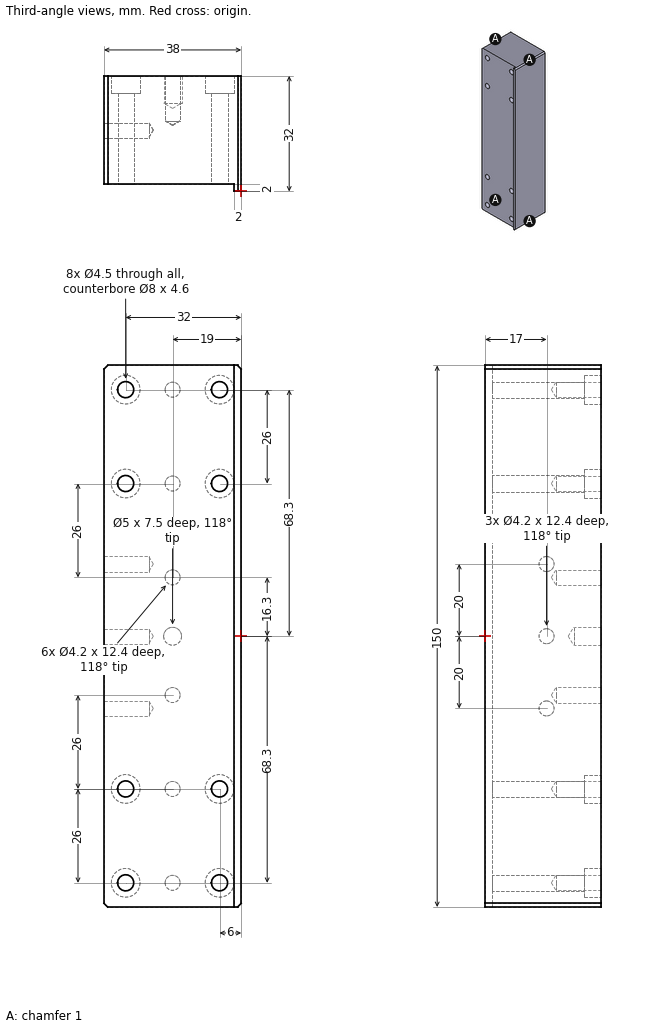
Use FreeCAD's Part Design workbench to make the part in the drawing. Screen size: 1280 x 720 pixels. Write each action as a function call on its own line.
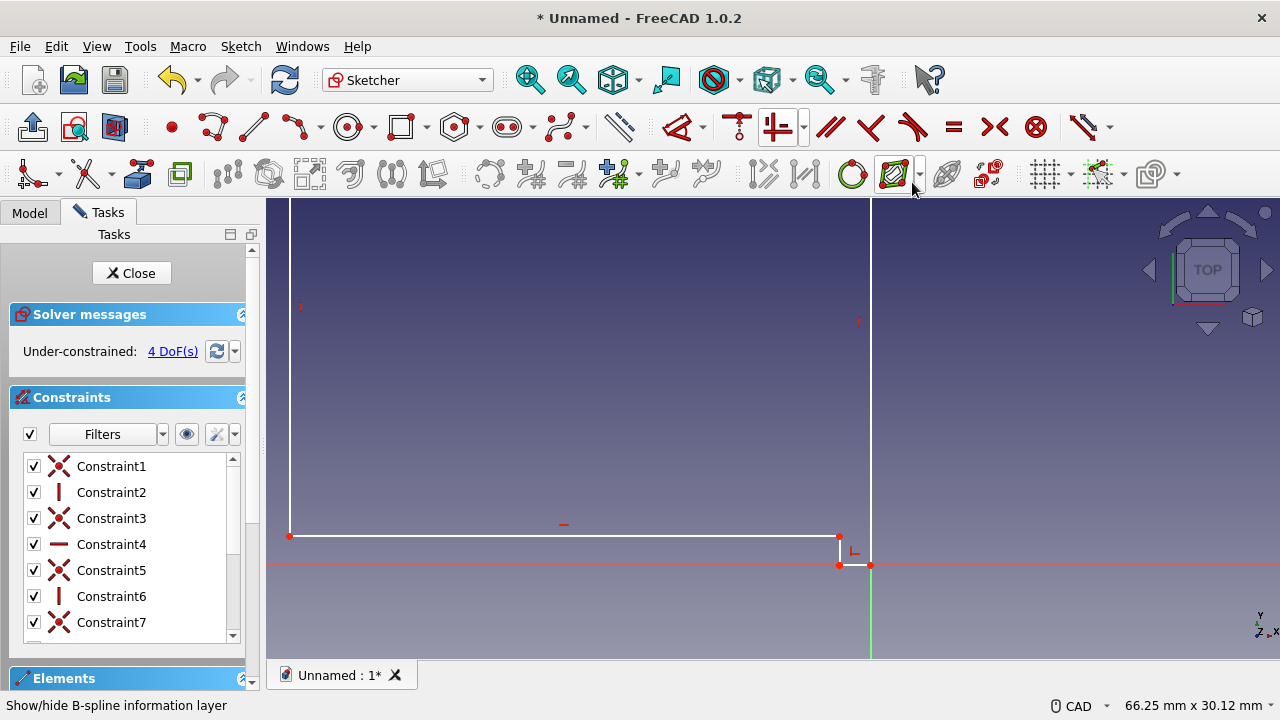
key(d)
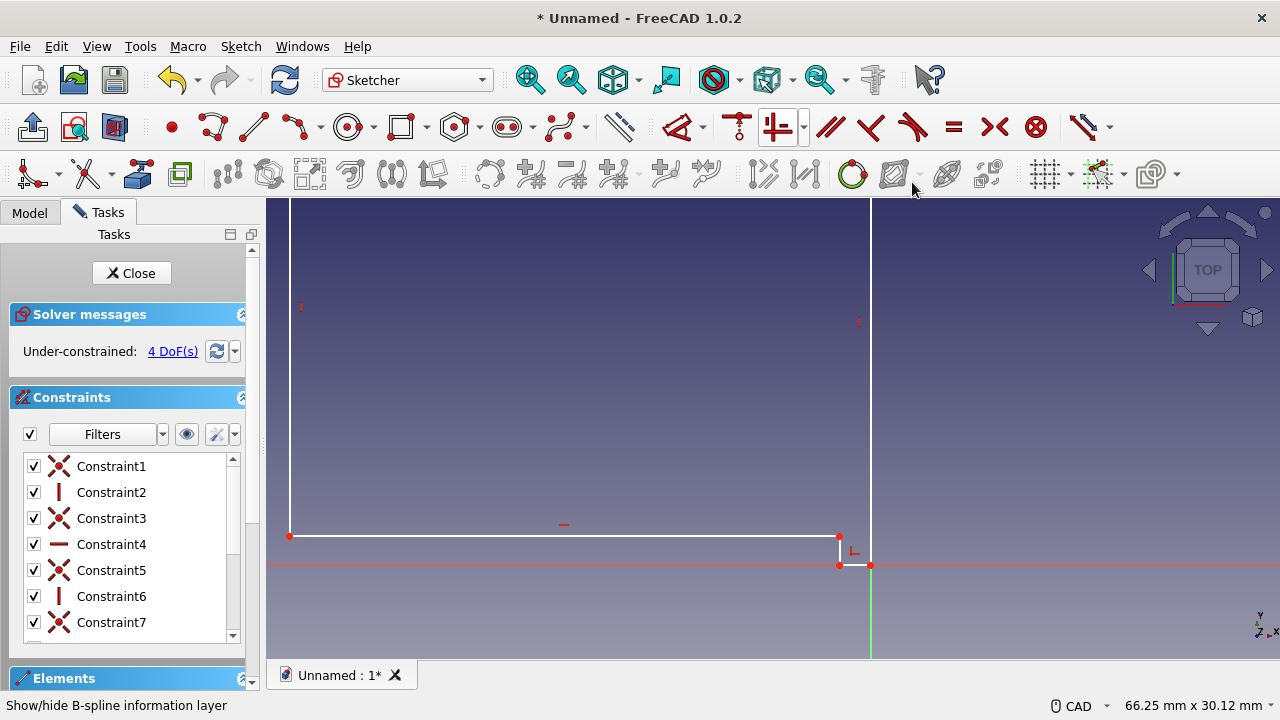
scroll(840, 548, up, 2)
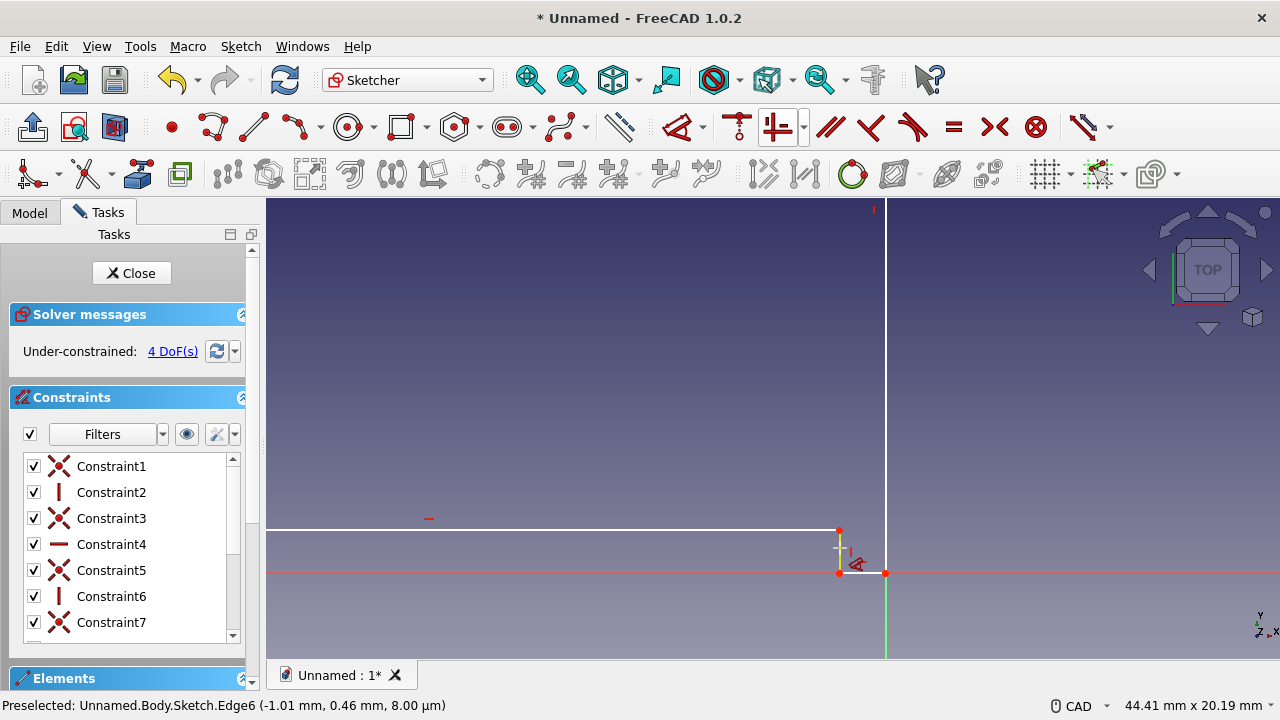
click(840, 548)
click(806, 552)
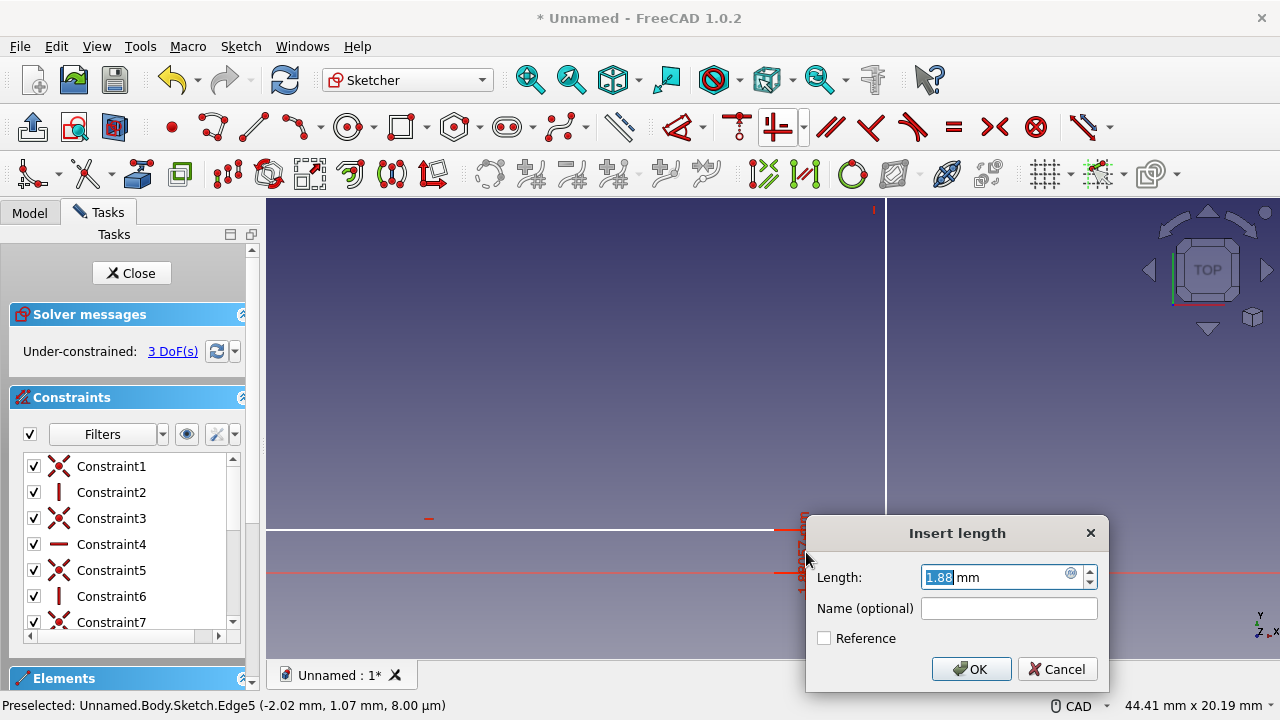
text(2)
key(Return)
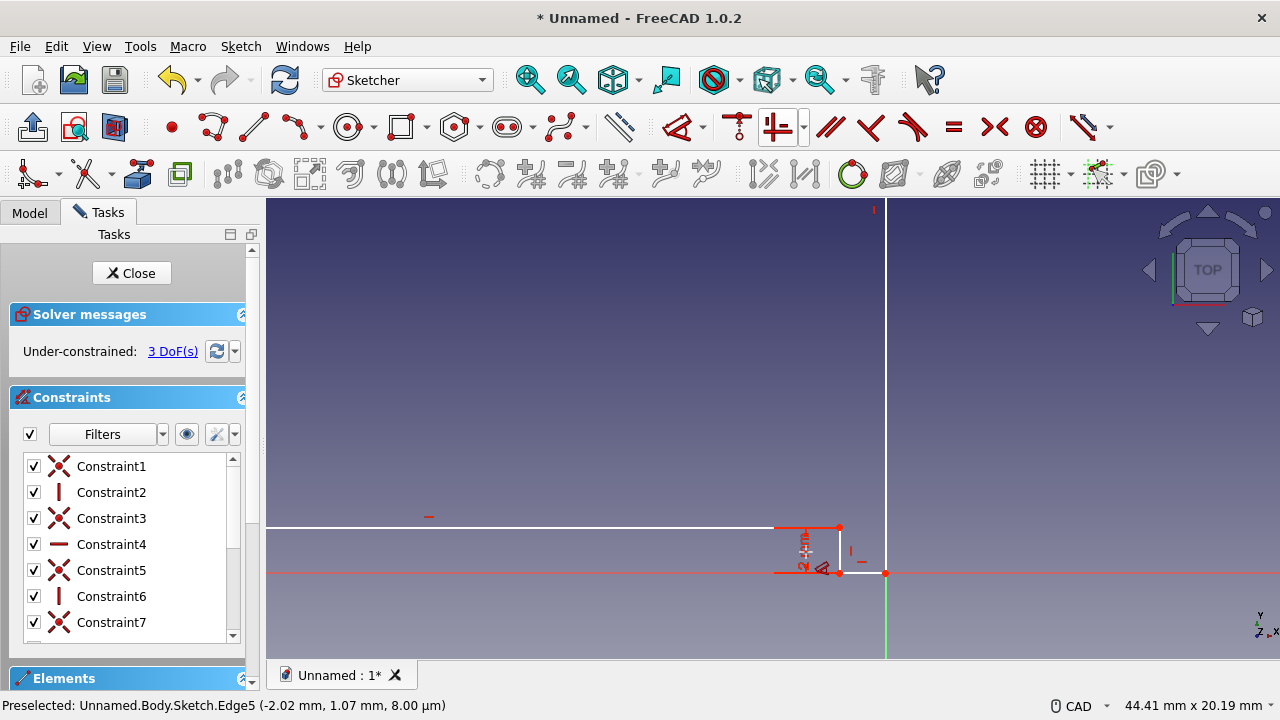
click(853, 573)
click(863, 607)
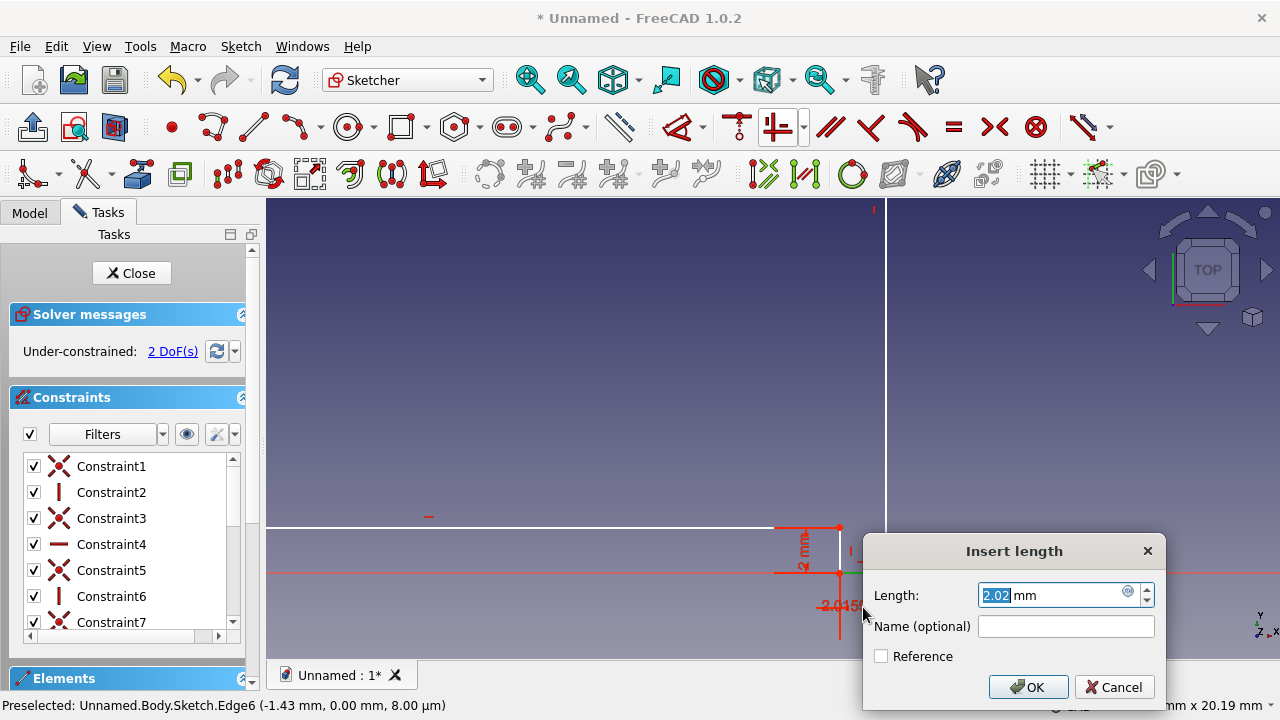
text(2)
key(Return)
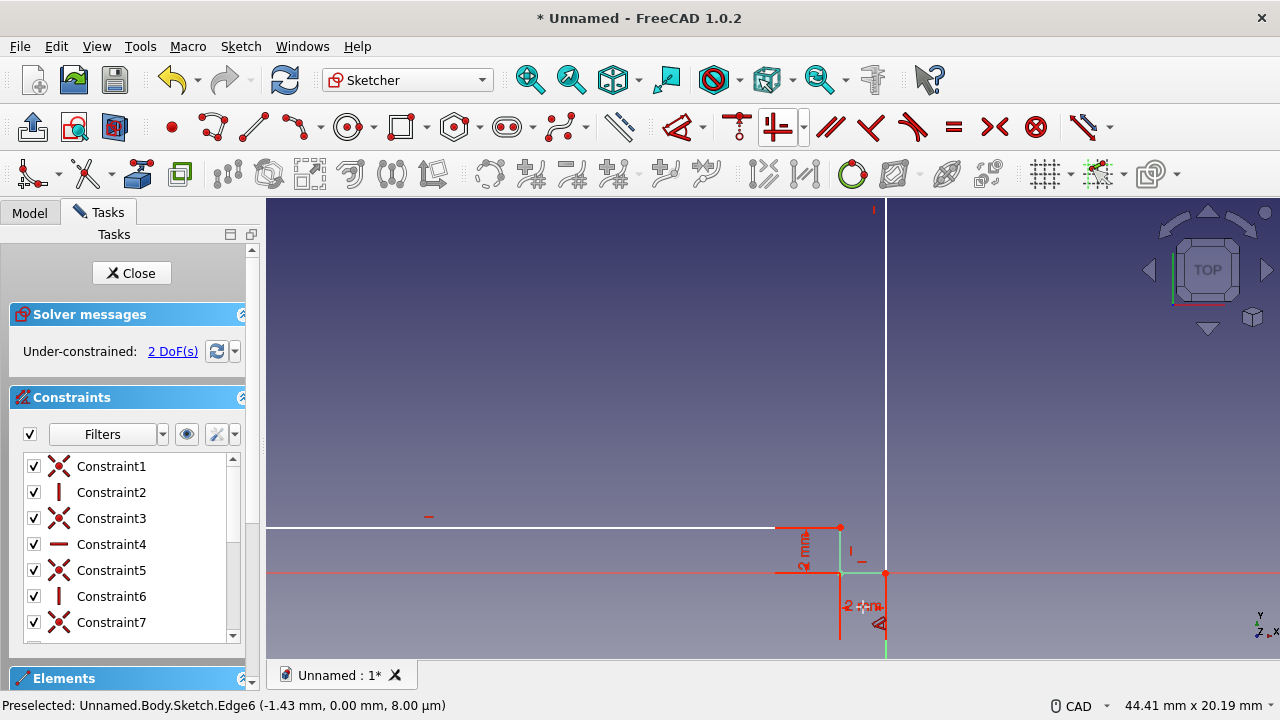
click(886, 355)
click(920, 400)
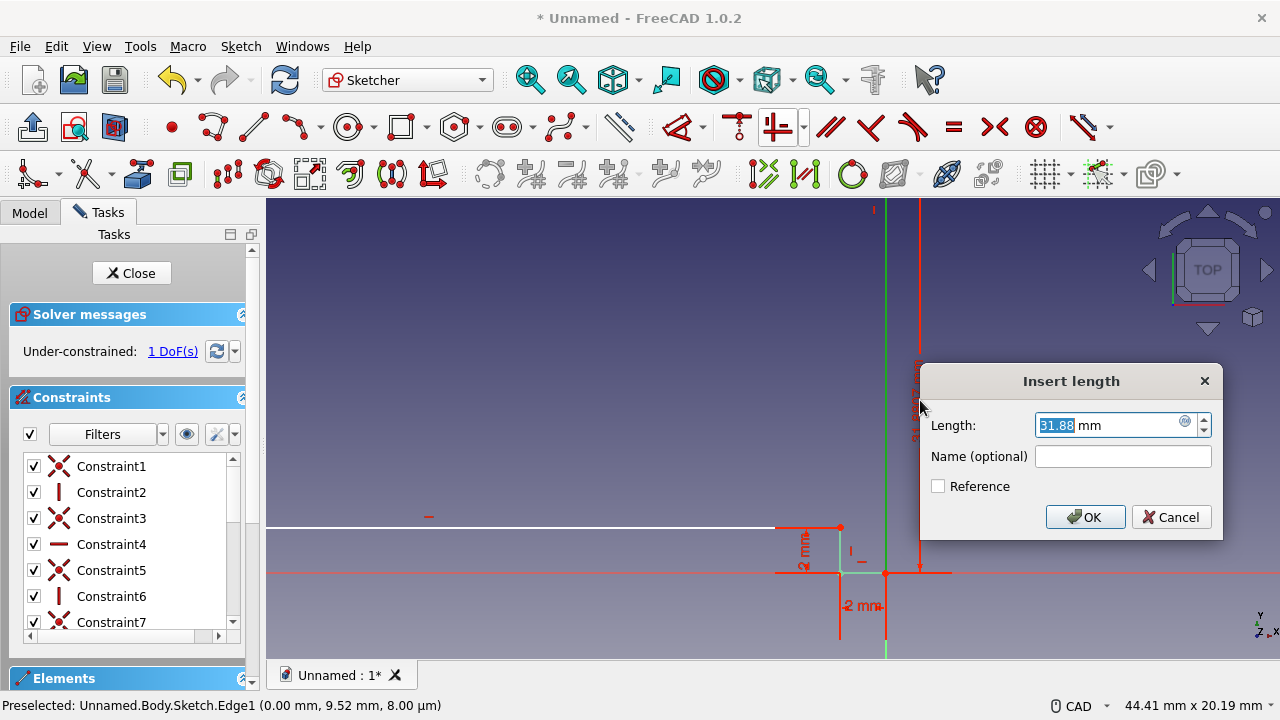
text(32)
key(Return)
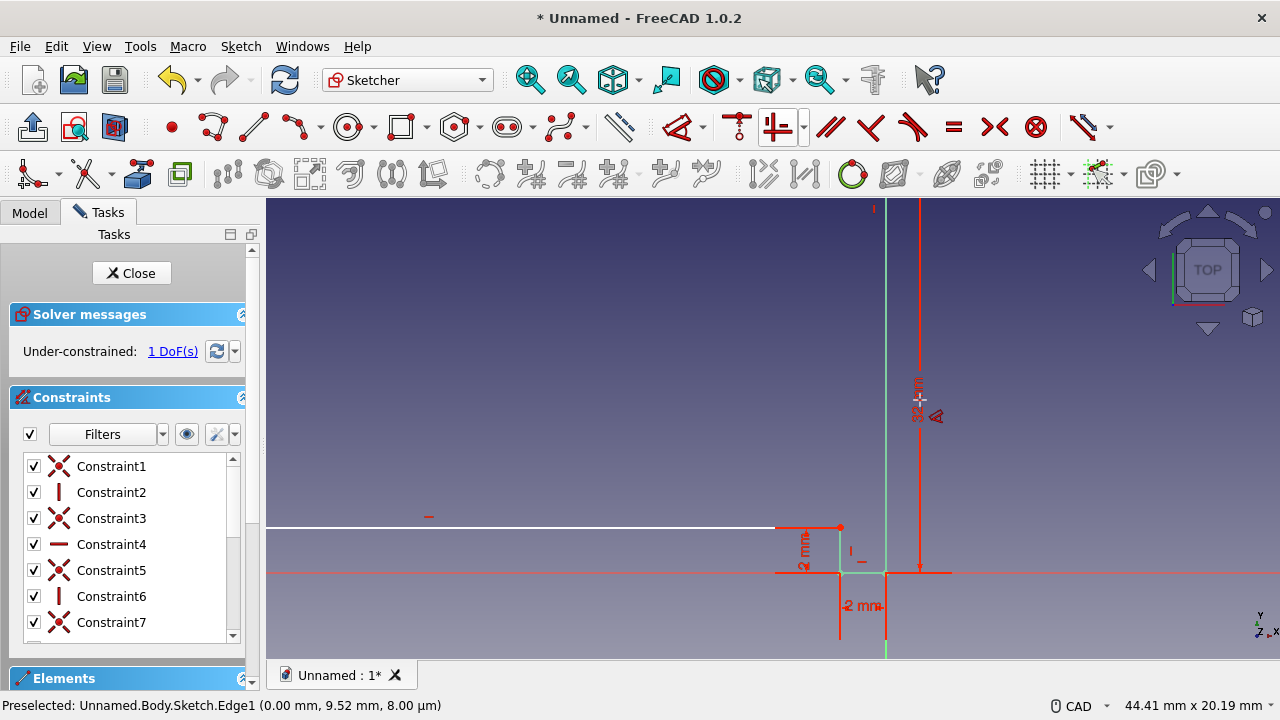
scroll(852, 557, down, 5)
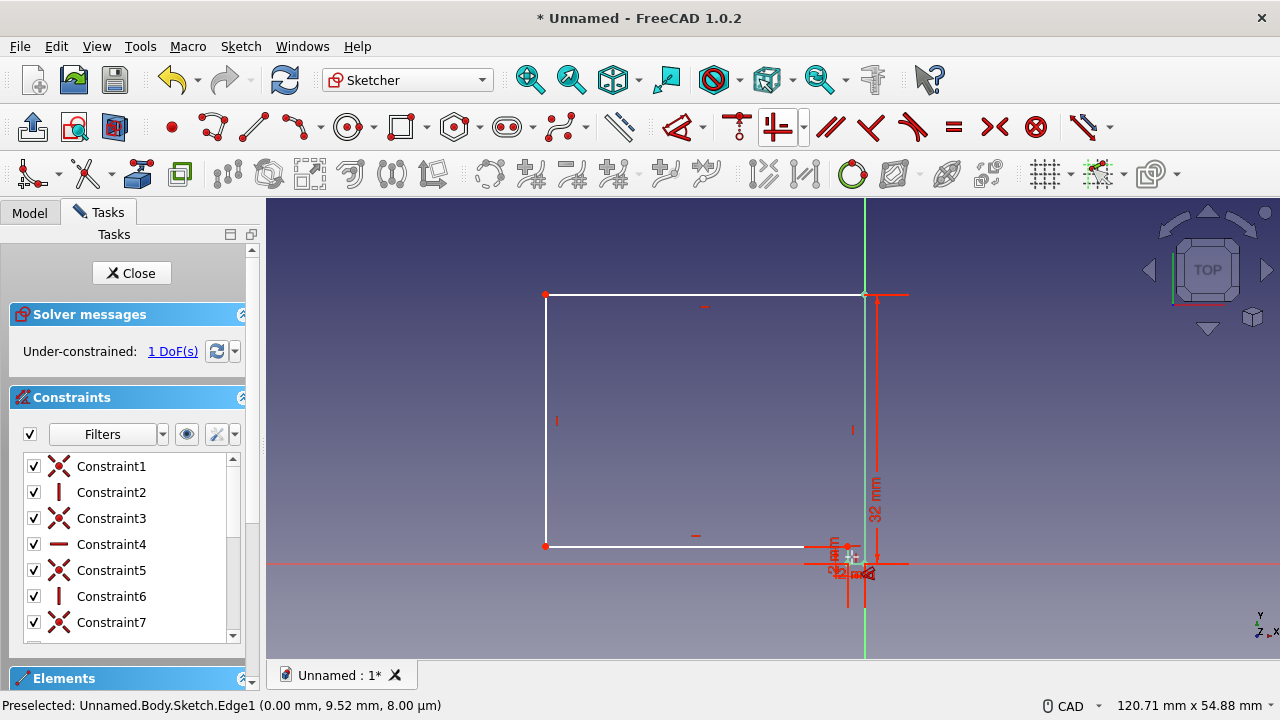
click(769, 295)
click(705, 261)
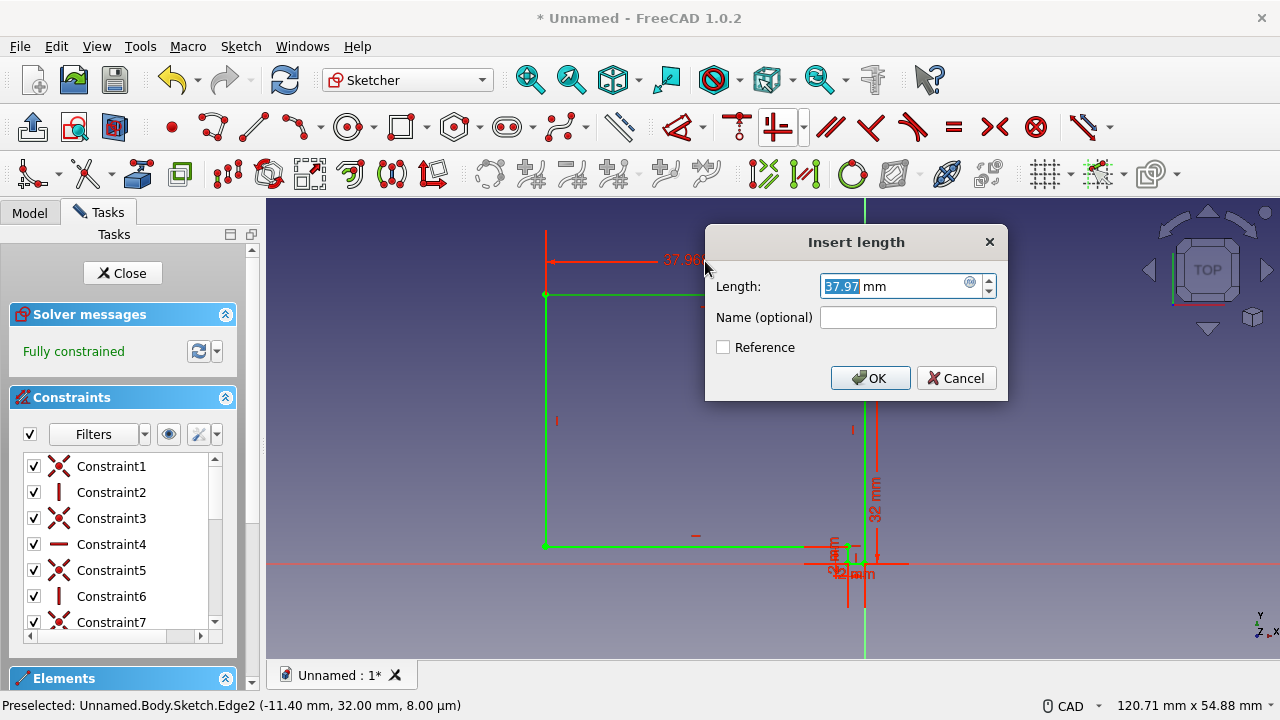
text(38)
key(Return)
key(Escape)